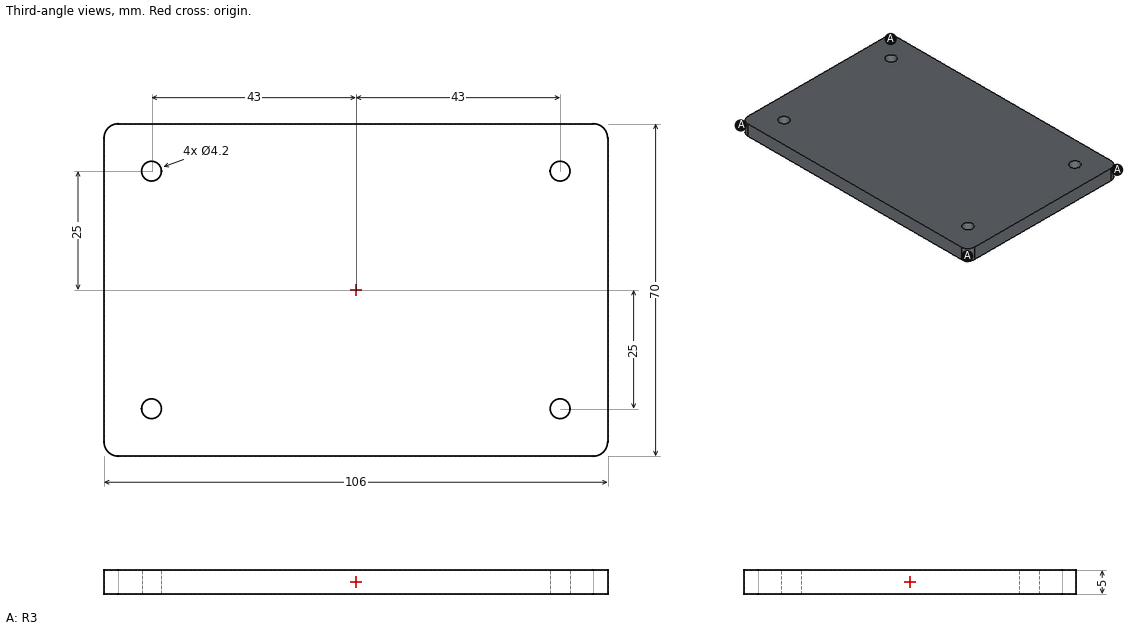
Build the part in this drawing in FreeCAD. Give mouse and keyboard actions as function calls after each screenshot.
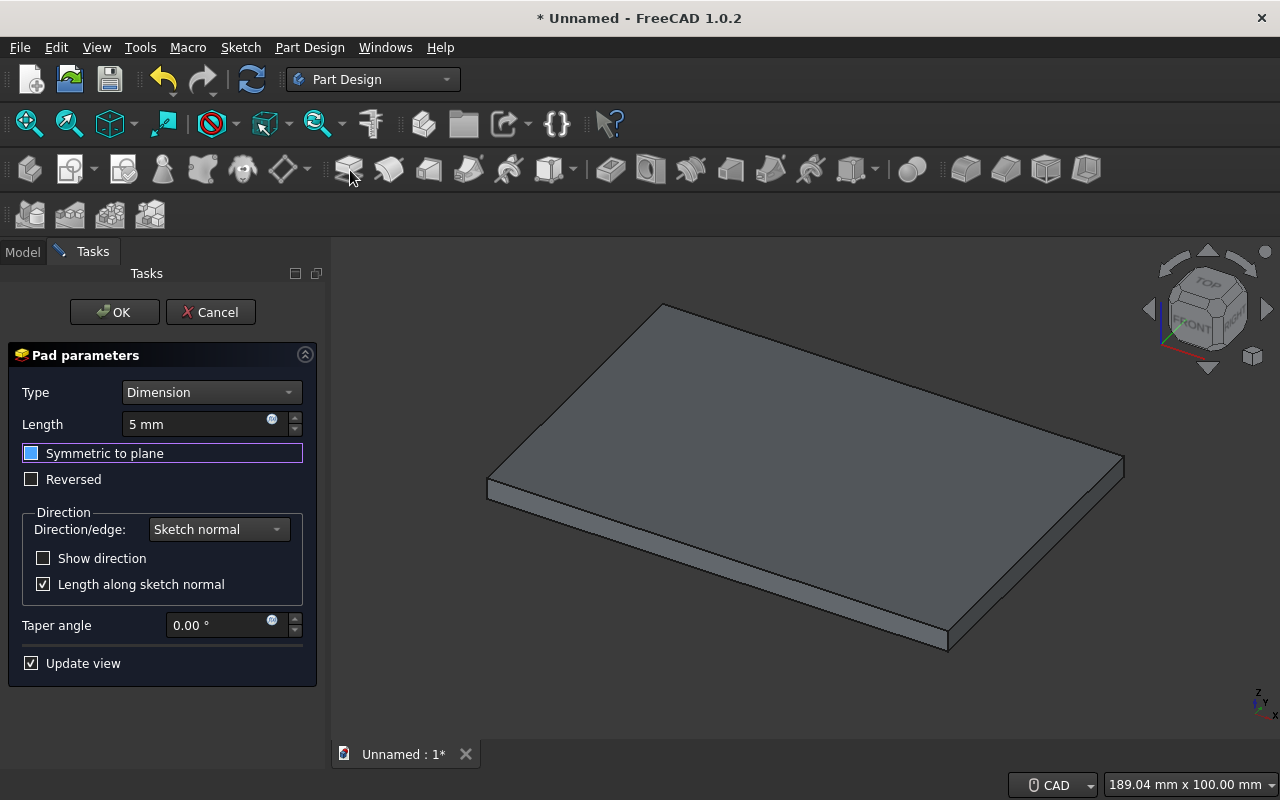
click(30, 453)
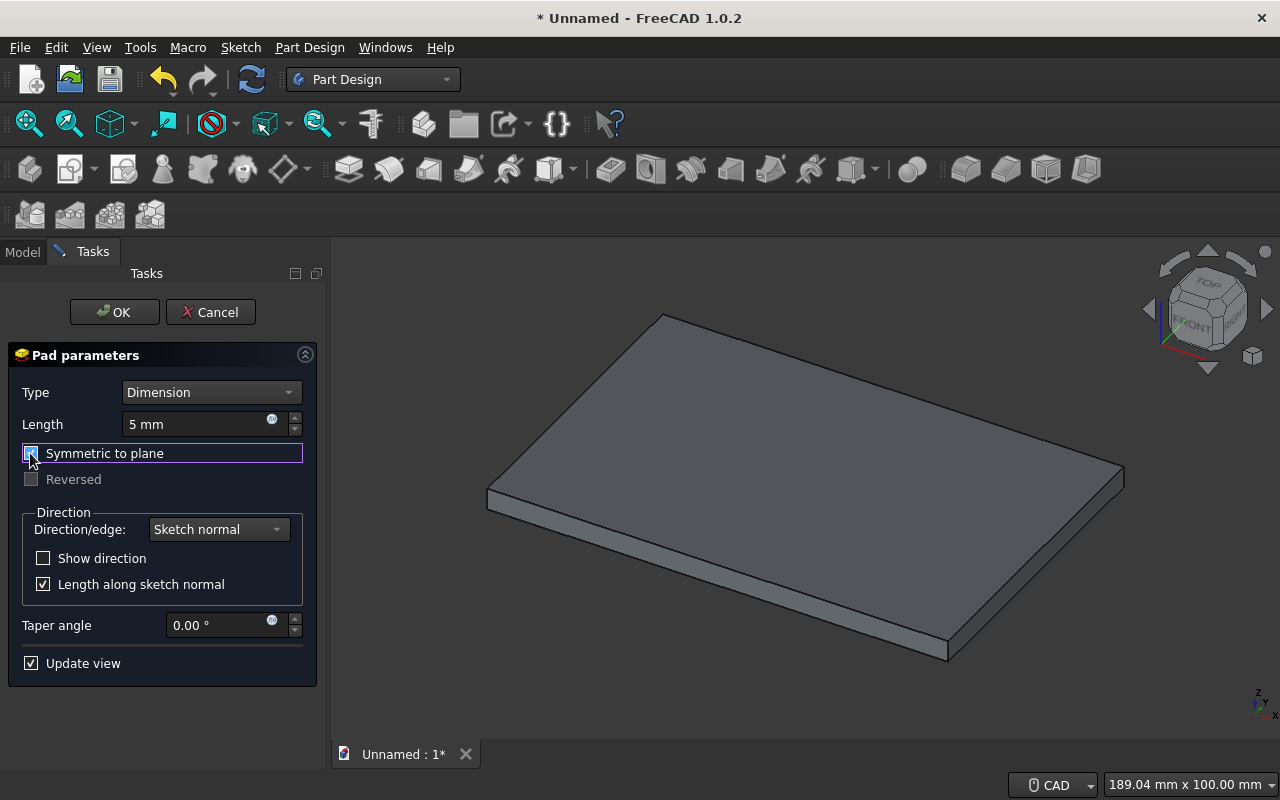
click(115, 312)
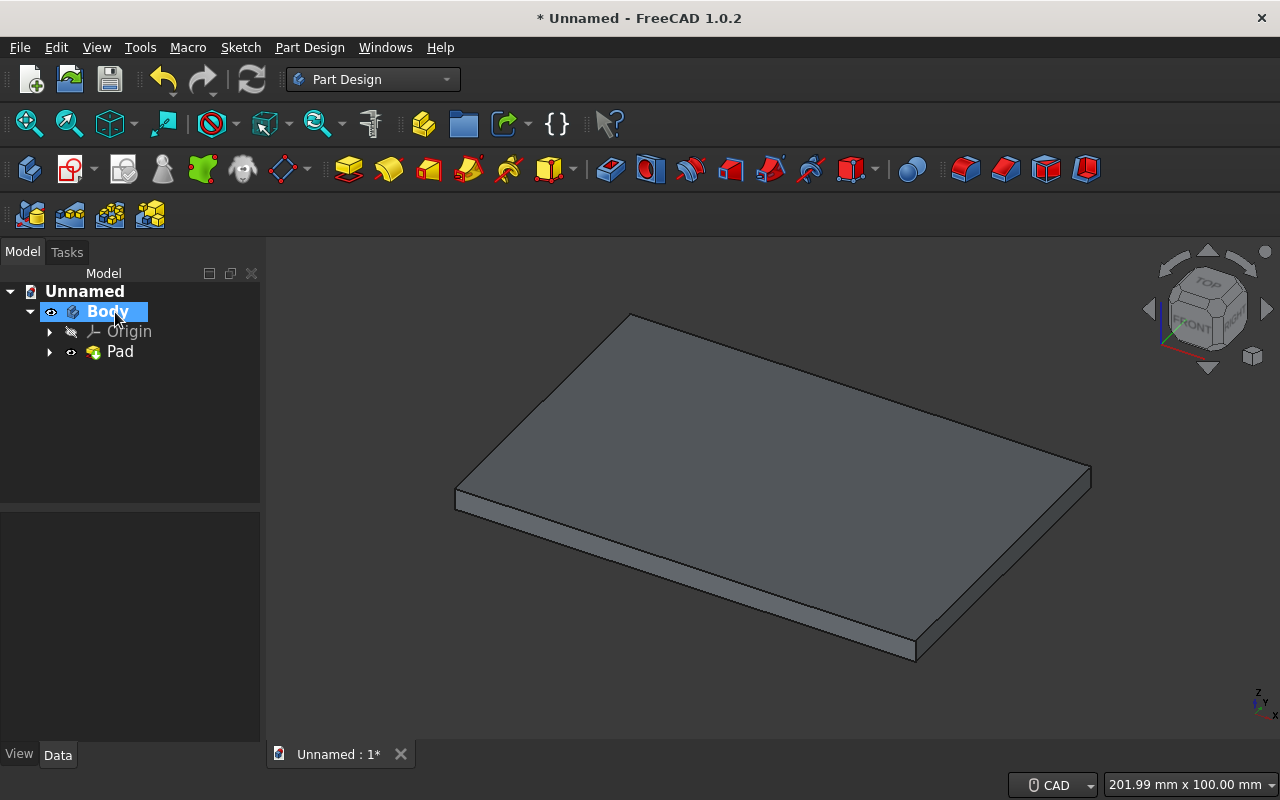
click(839, 499)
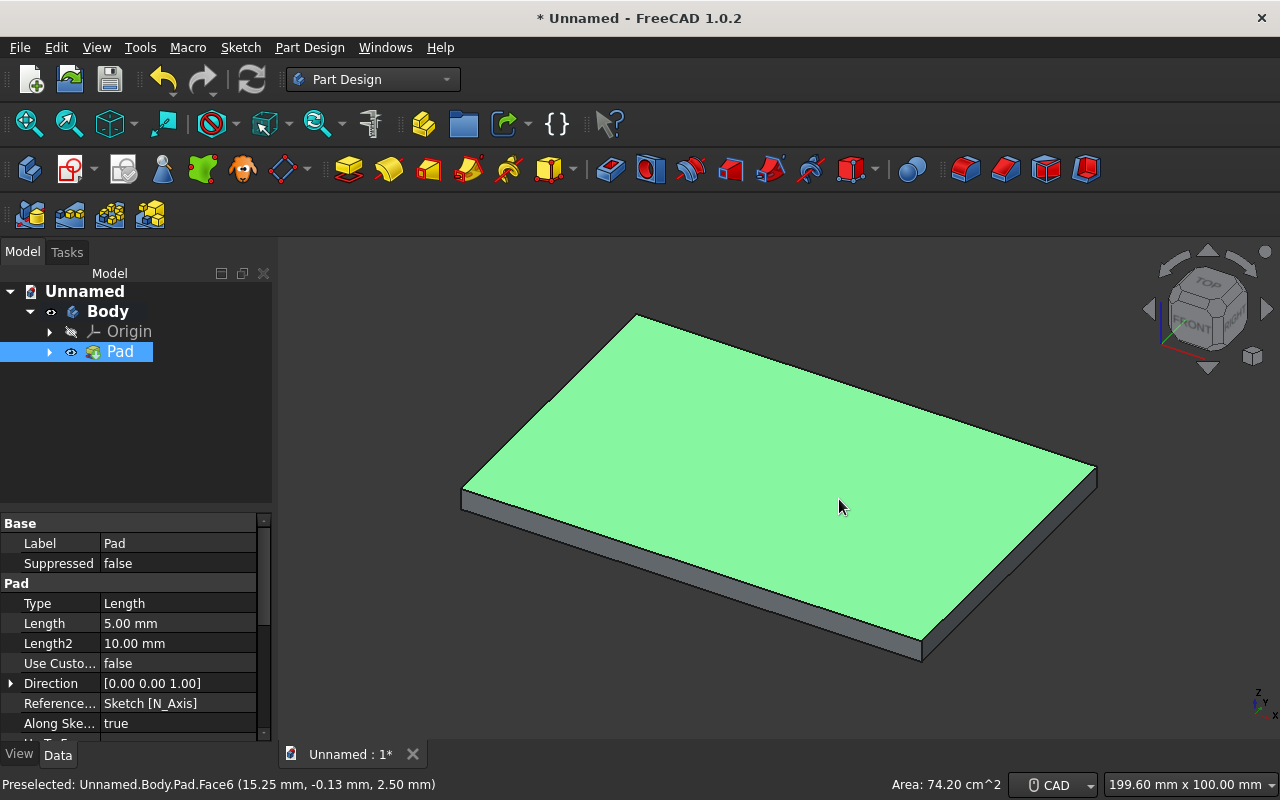
click(70, 170)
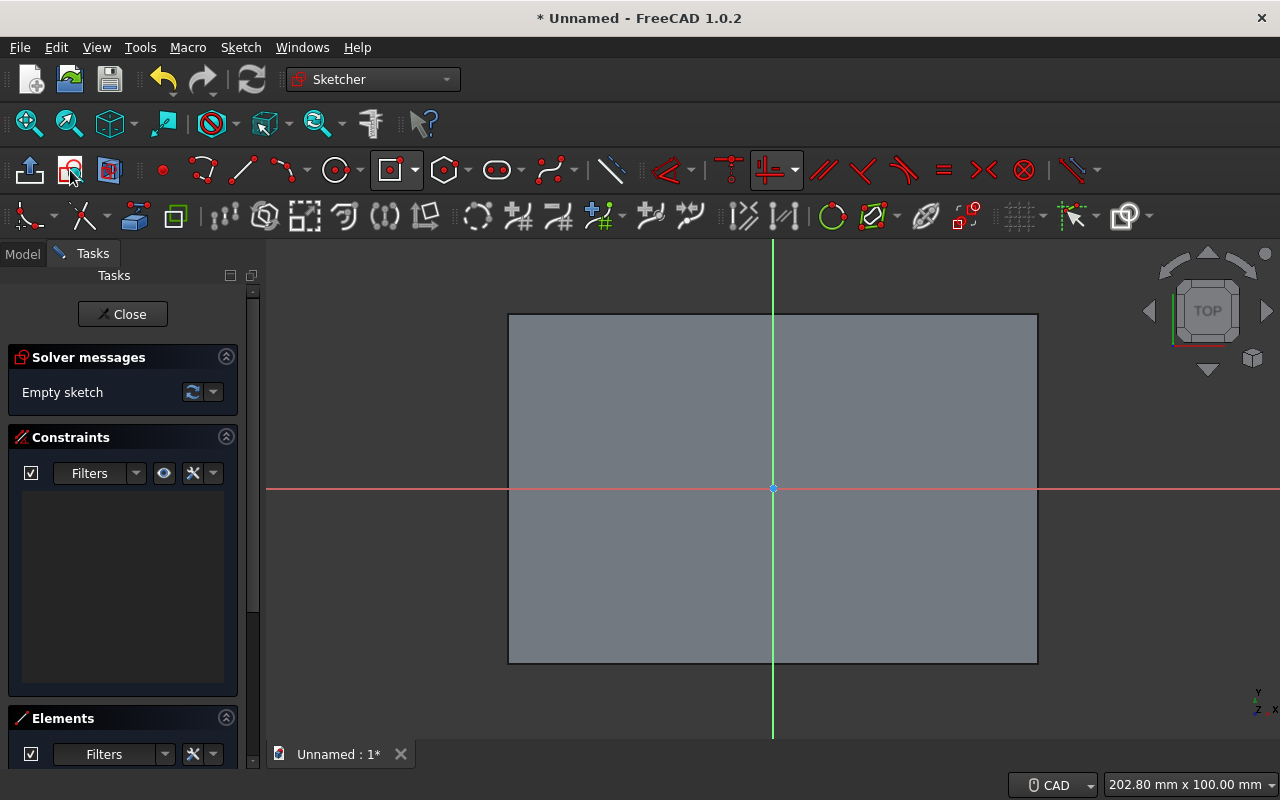
click(336, 170)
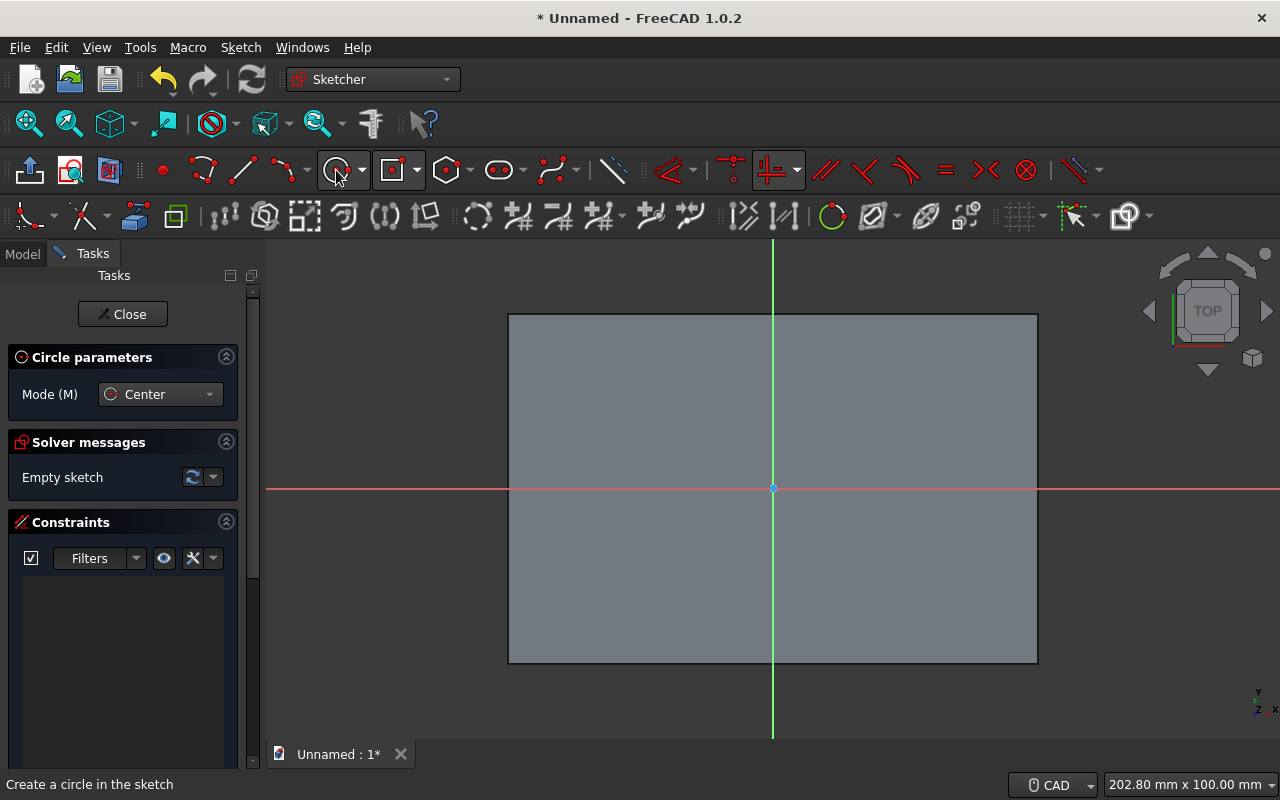
scroll(558, 364, up, 4)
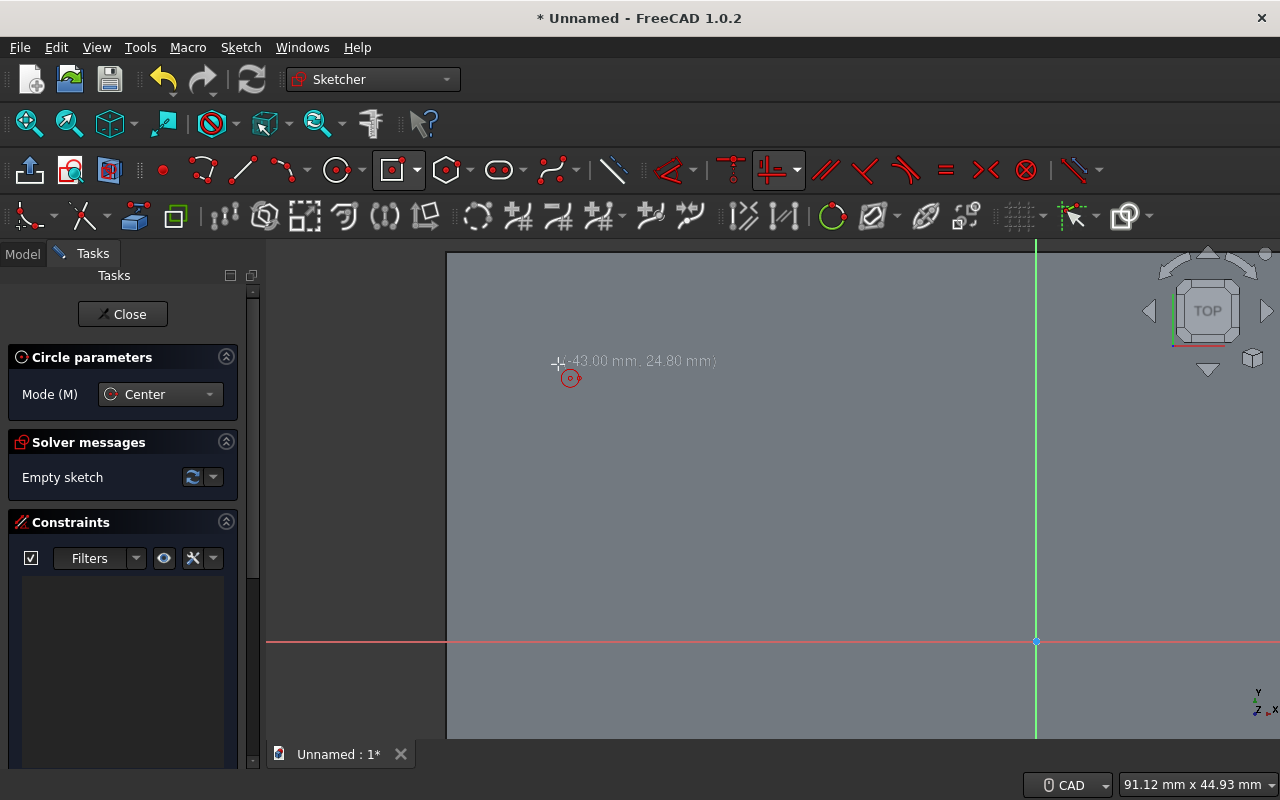
click(558, 364)
move(574, 347)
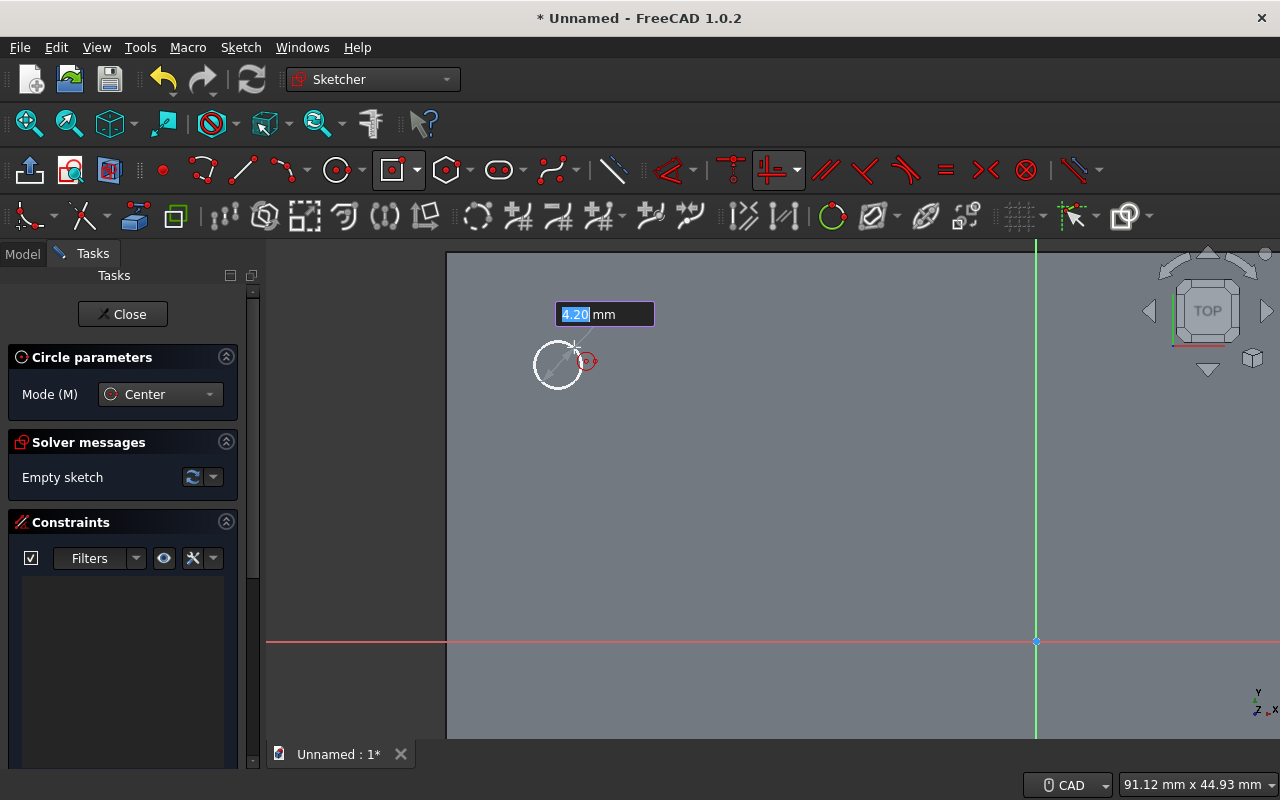
text(4.2)
key(Return)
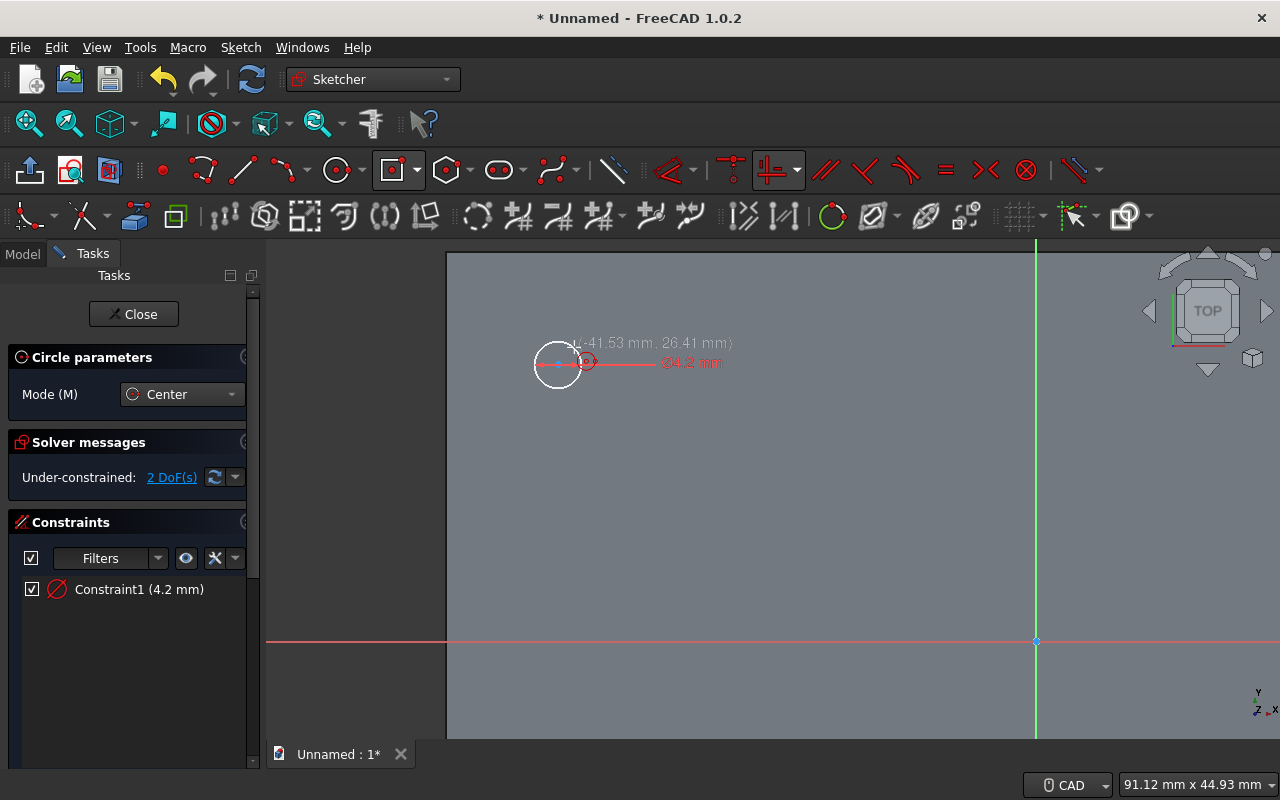
scroll(301, 303, down, 3)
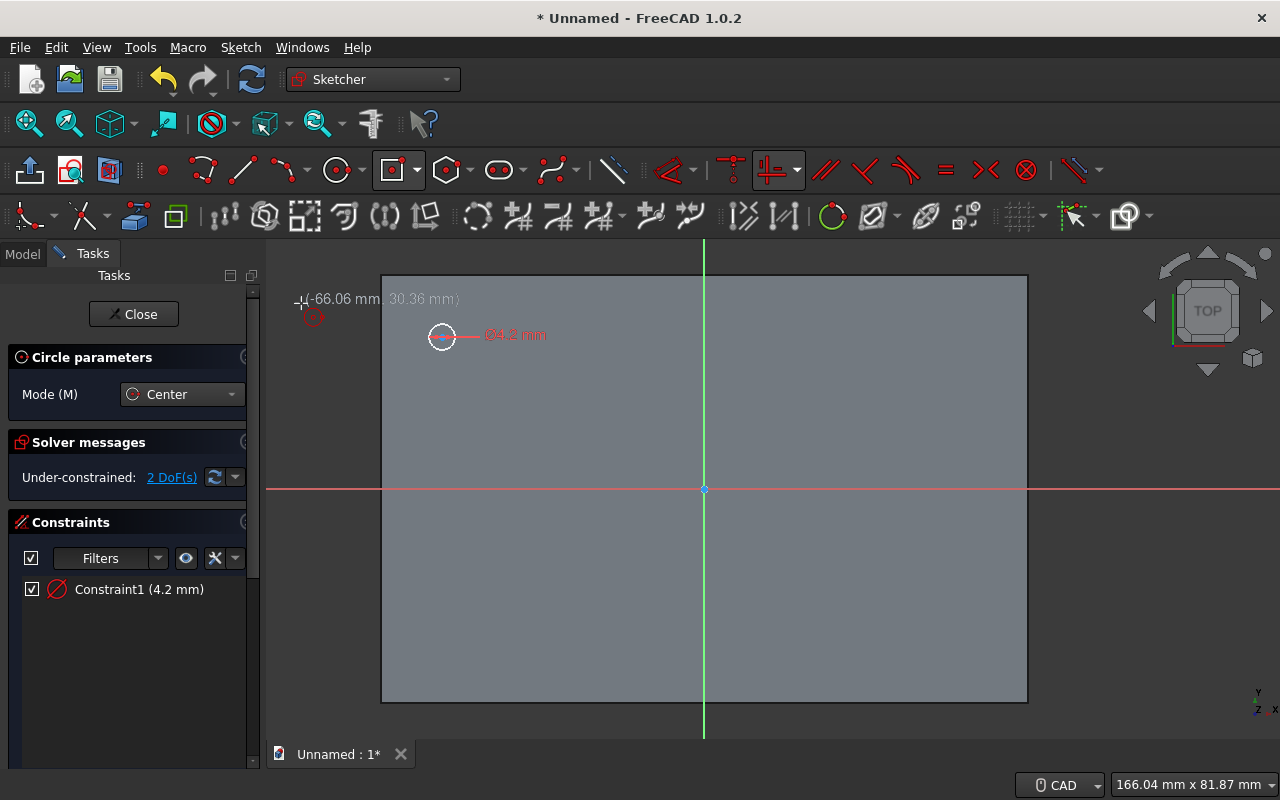
scroll(967, 336, up, 3)